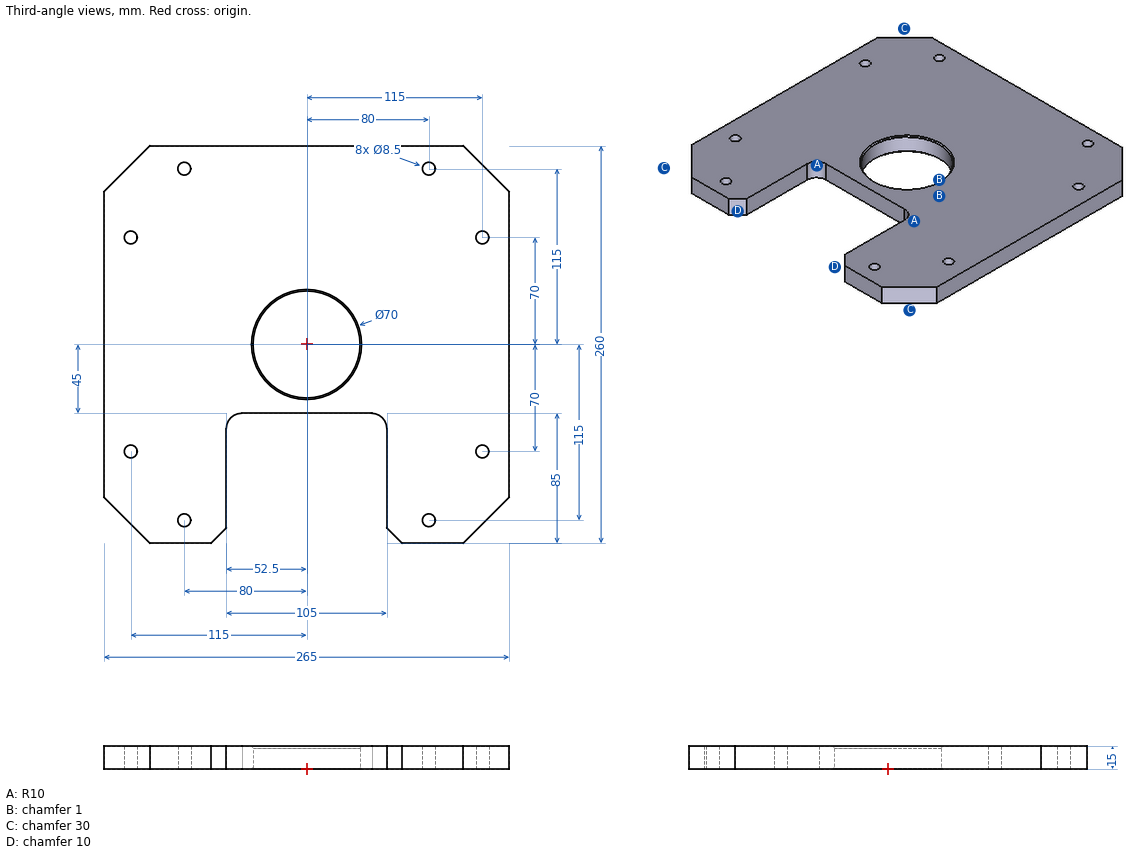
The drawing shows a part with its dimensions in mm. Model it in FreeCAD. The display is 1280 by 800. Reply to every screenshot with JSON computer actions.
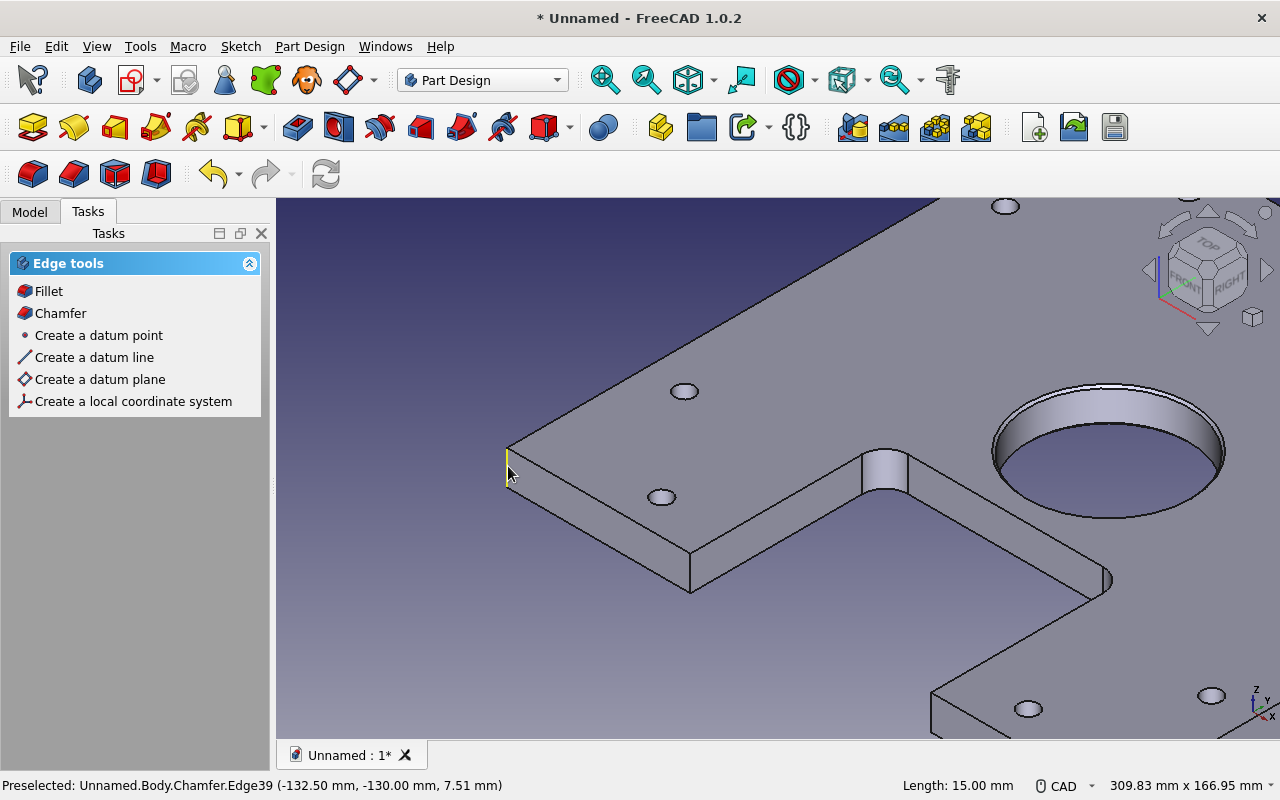
{"action": "left_click", "coordinate": [606, 80]}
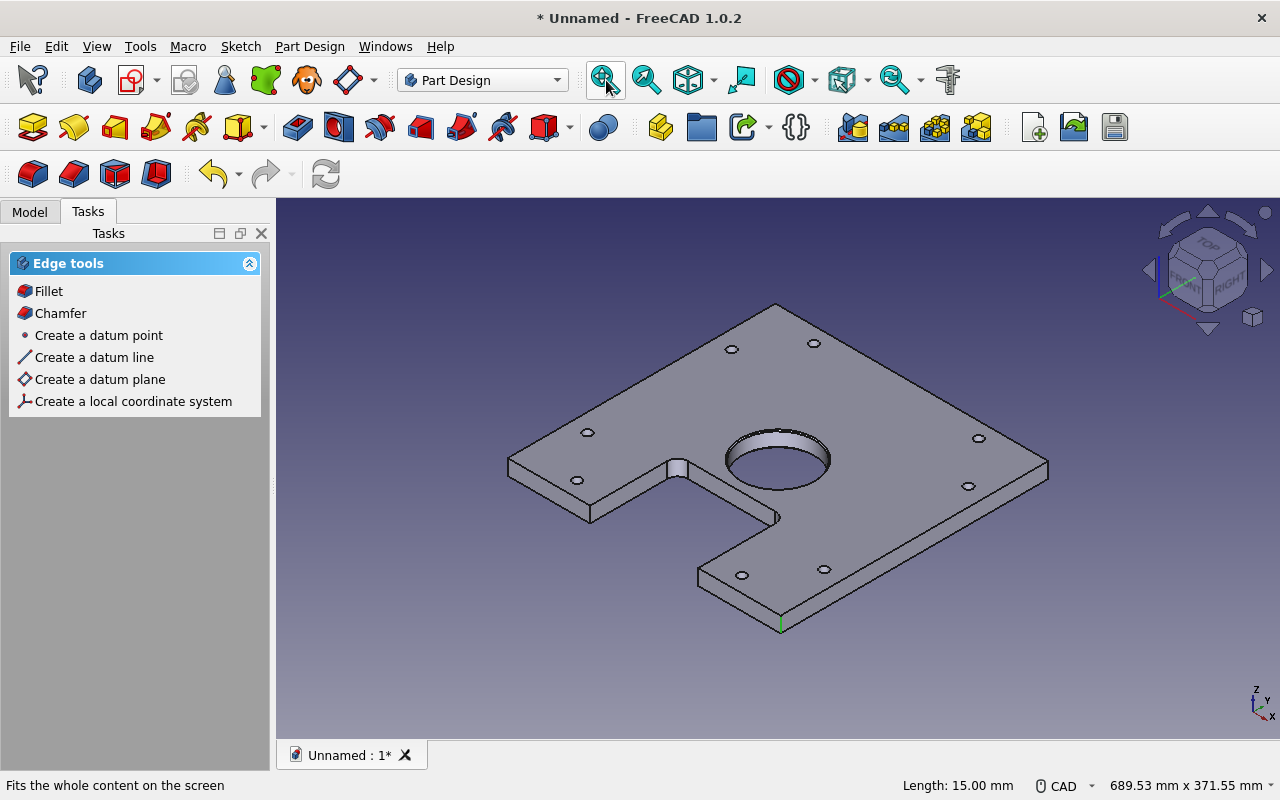
{"action": "key", "text": "2"}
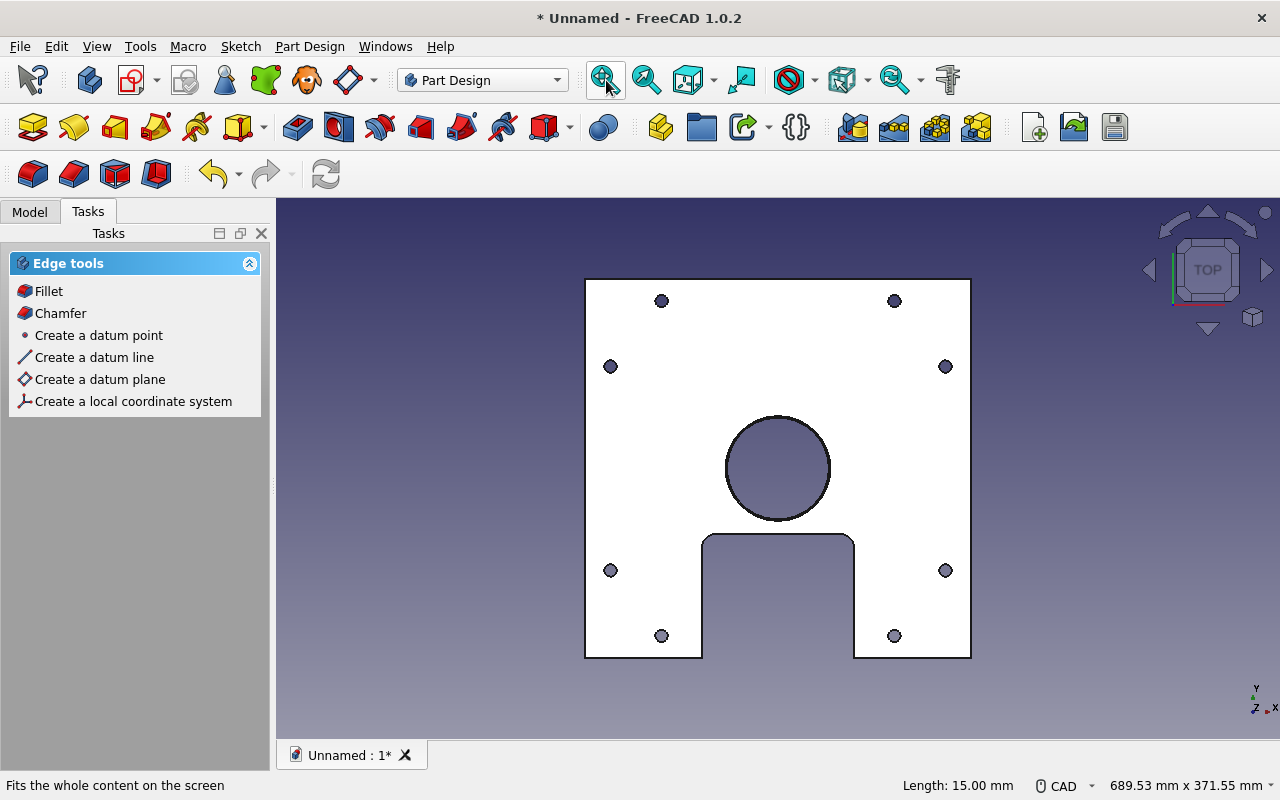
{"action": "scroll", "coordinate": [585, 657], "scroll_direction": "up", "scroll_amount": 4}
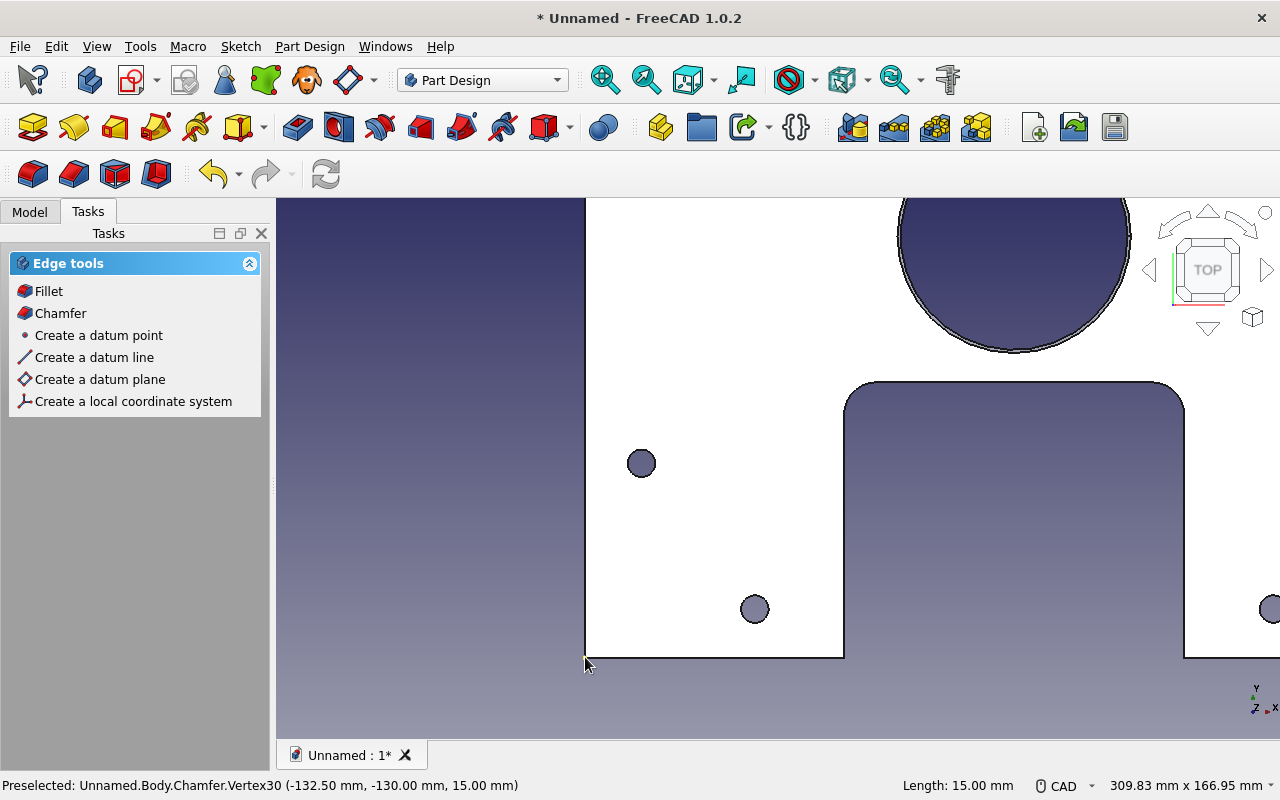
{"action": "left_click", "coordinate": [606, 80]}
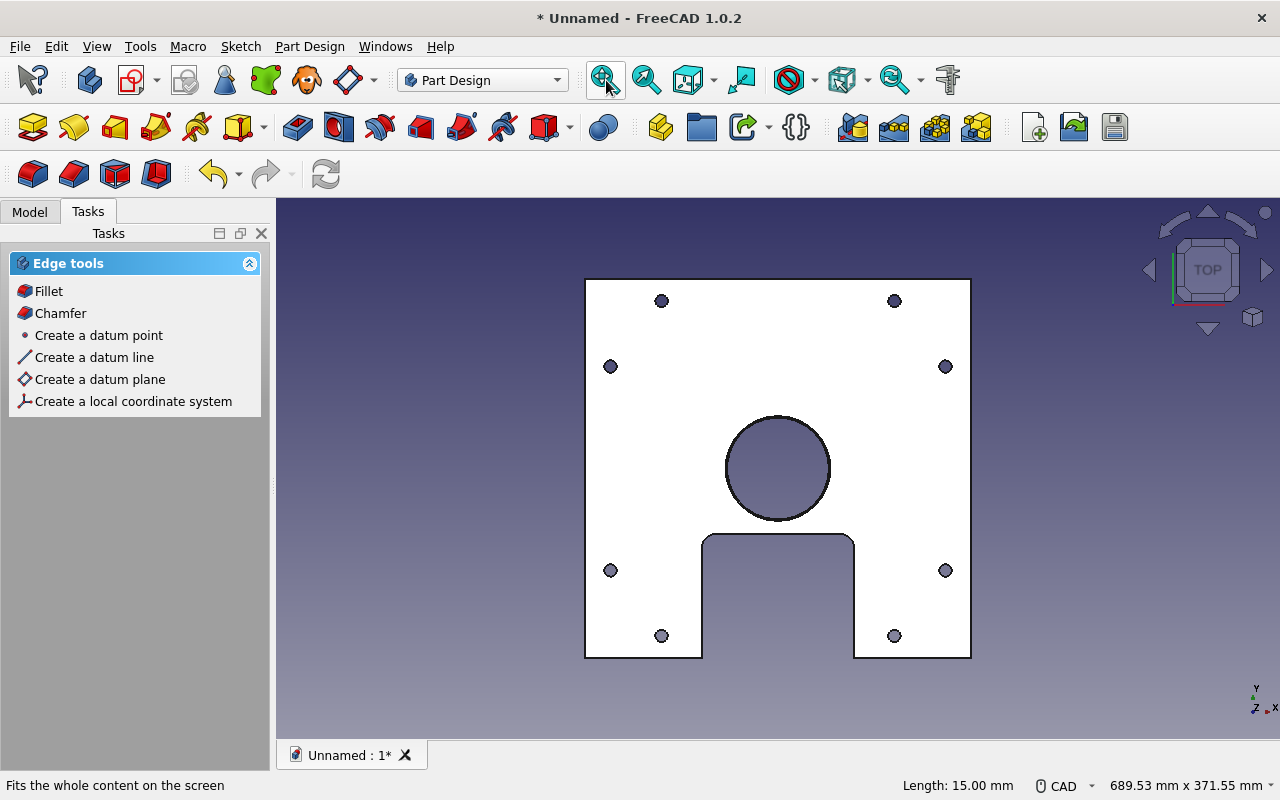
{"action": "key", "text": "1"}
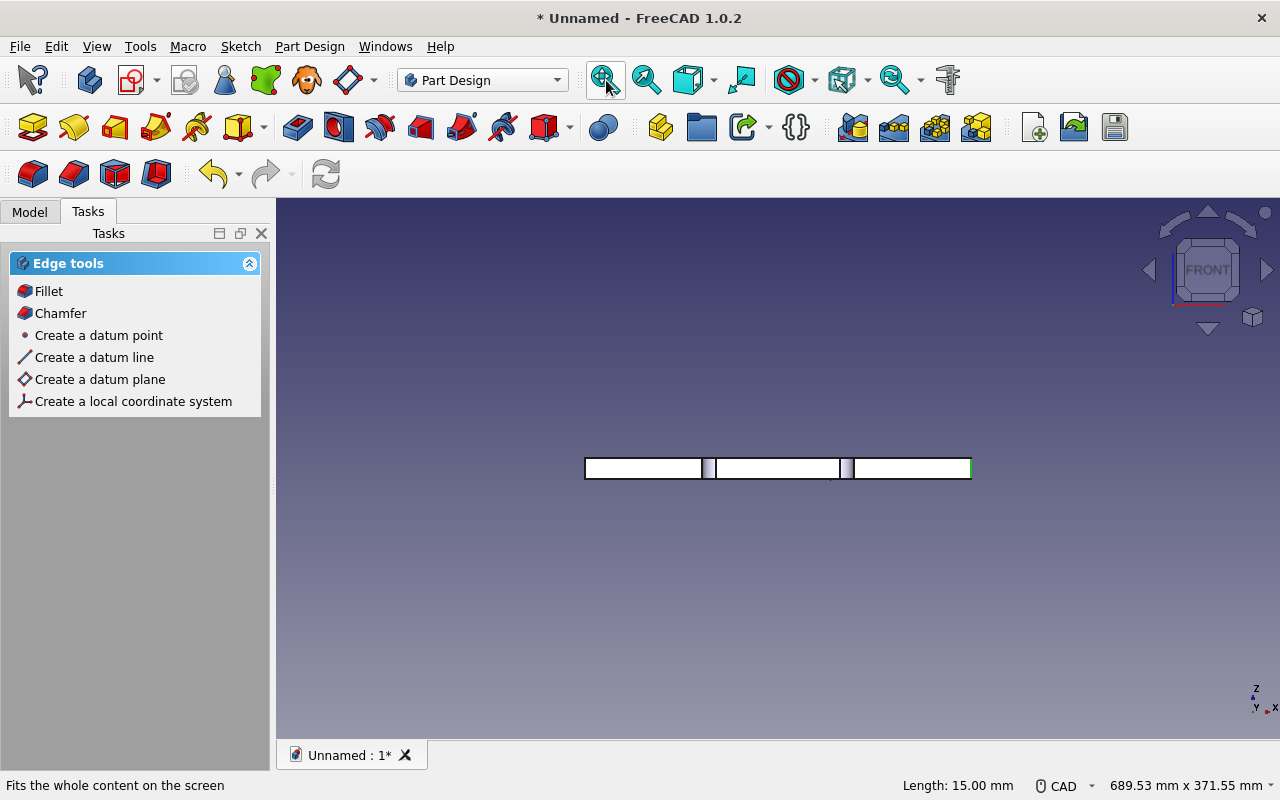
{"action": "left_click", "coordinate": [606, 80]}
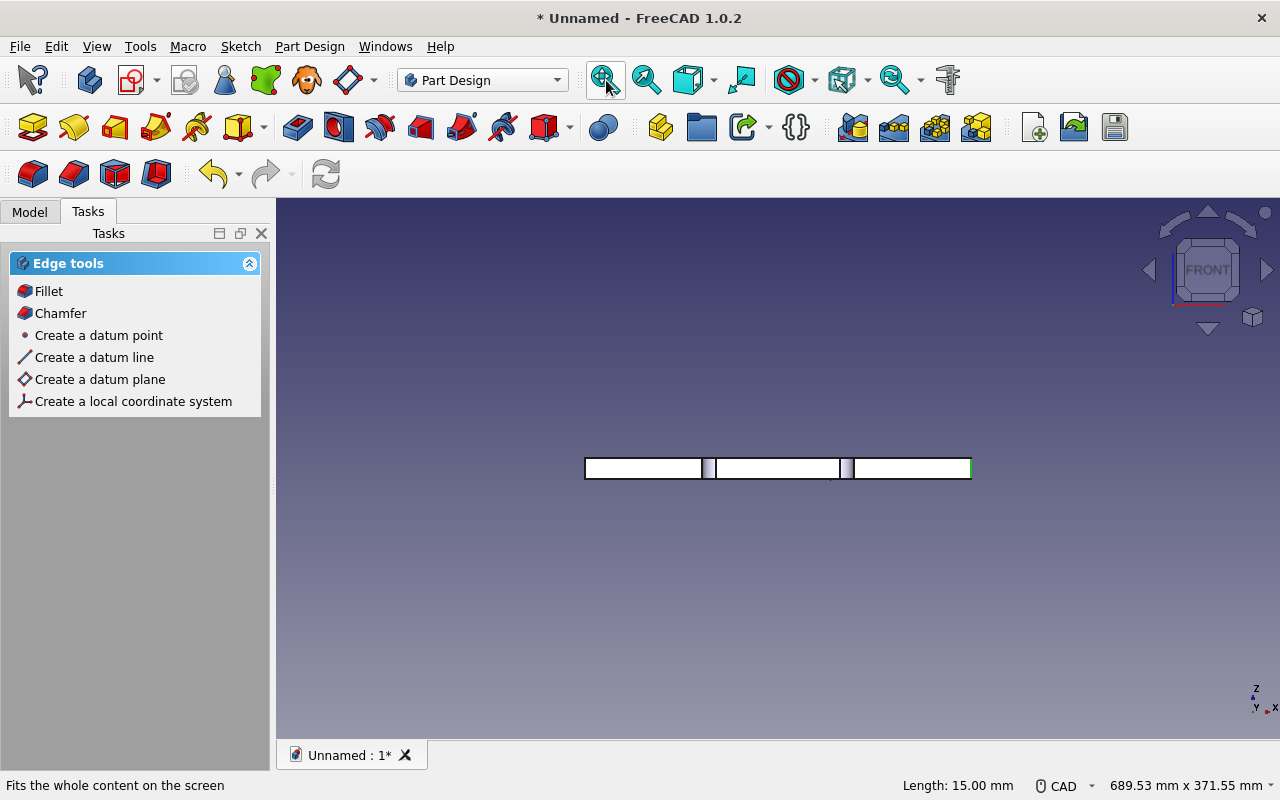
{"action": "left_click", "coordinate": [585, 468], "text": "ctrl"}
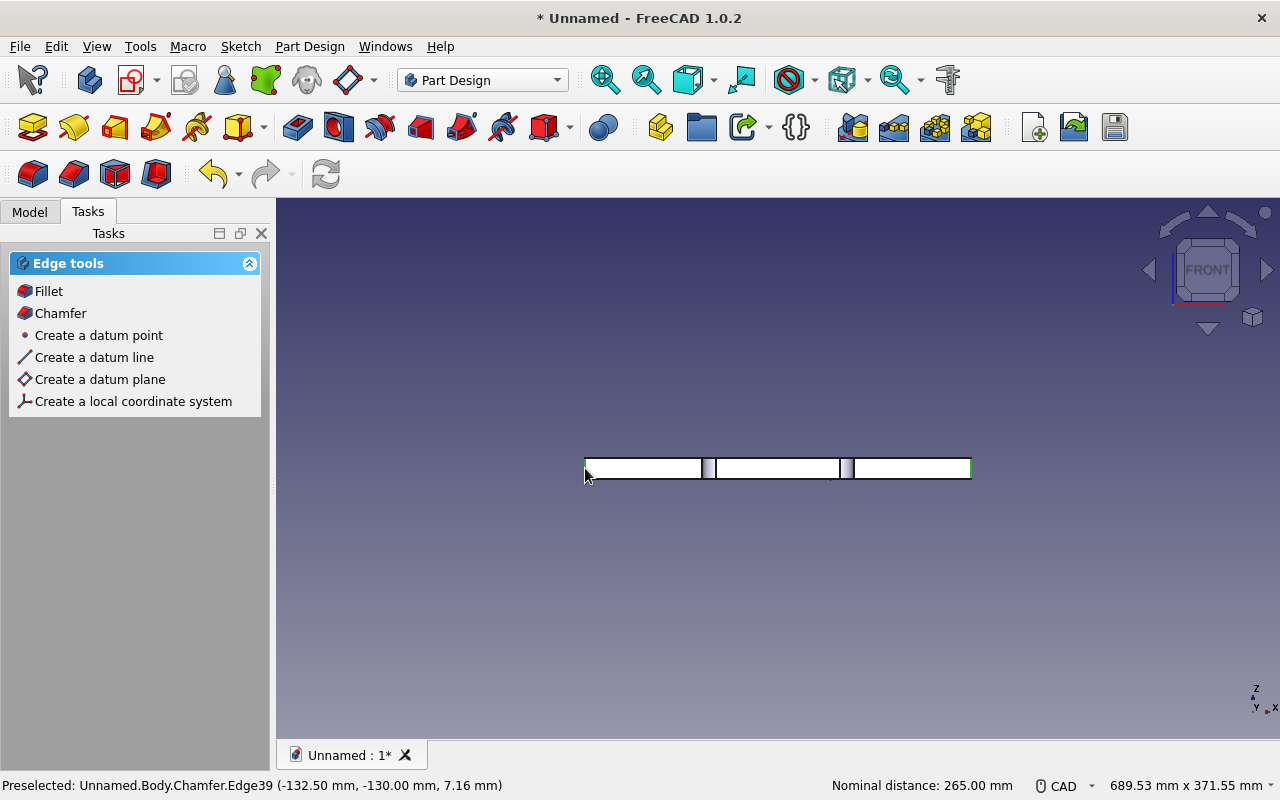
{"action": "scroll", "coordinate": [585, 468], "scroll_direction": "up", "scroll_amount": 4}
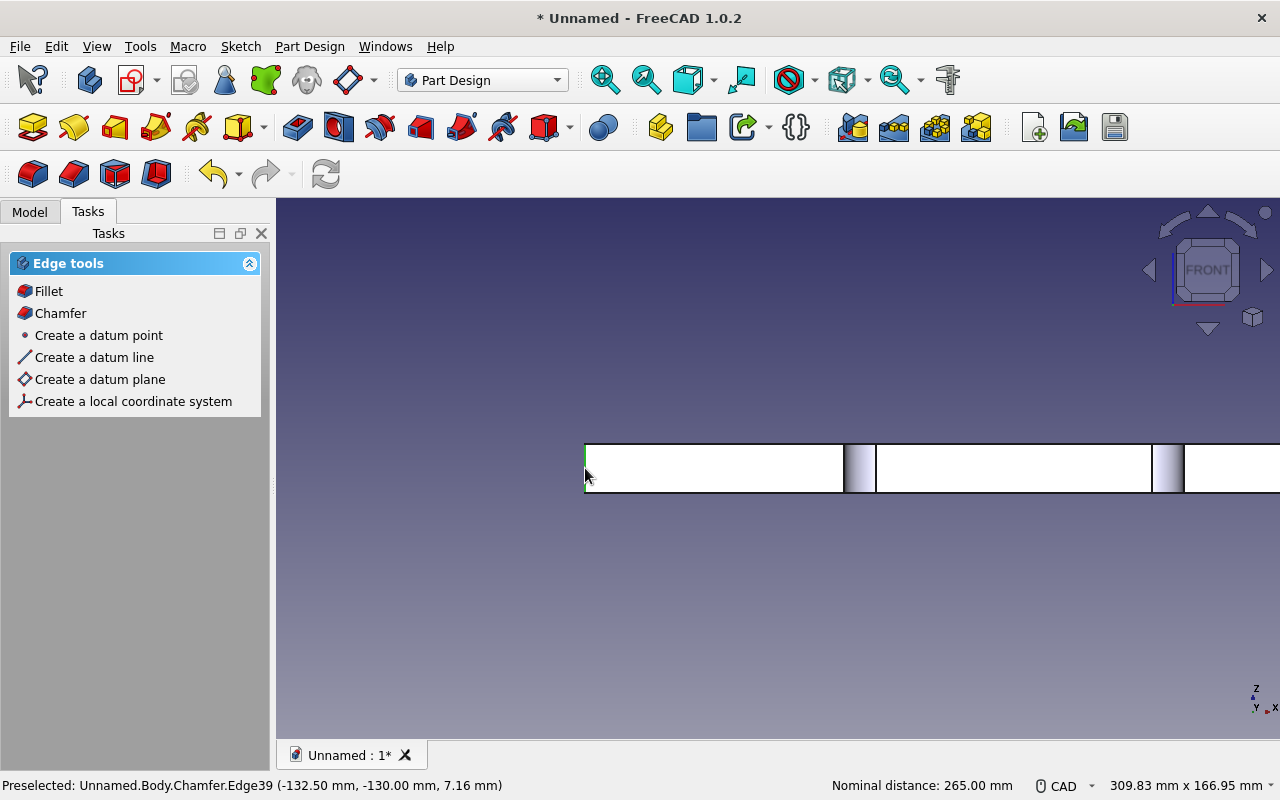
{"action": "key", "text": "v f"}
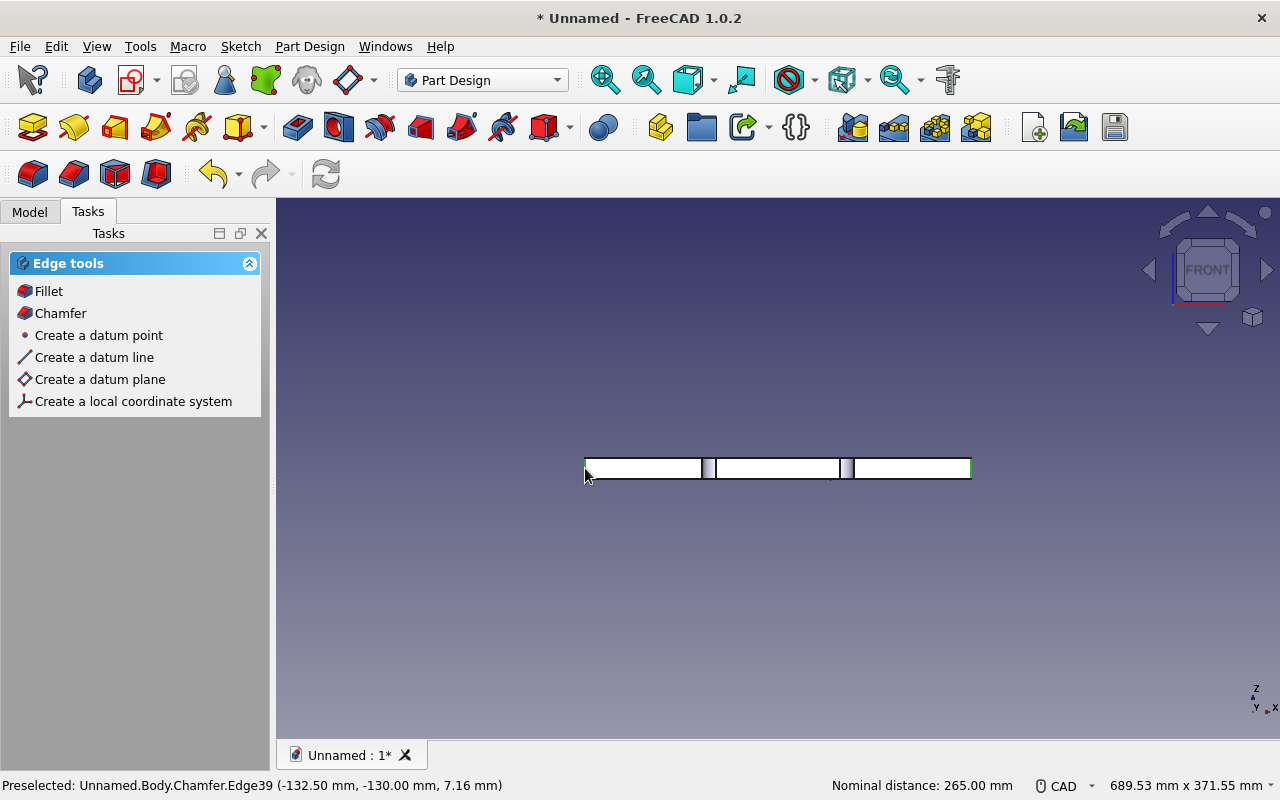
{"action": "key", "text": "3"}